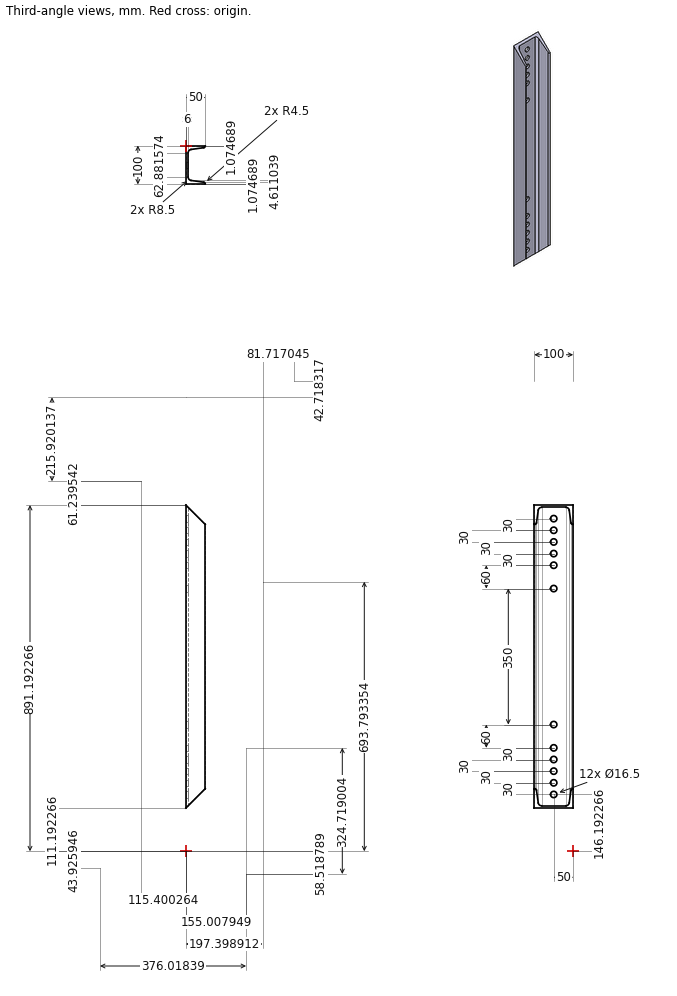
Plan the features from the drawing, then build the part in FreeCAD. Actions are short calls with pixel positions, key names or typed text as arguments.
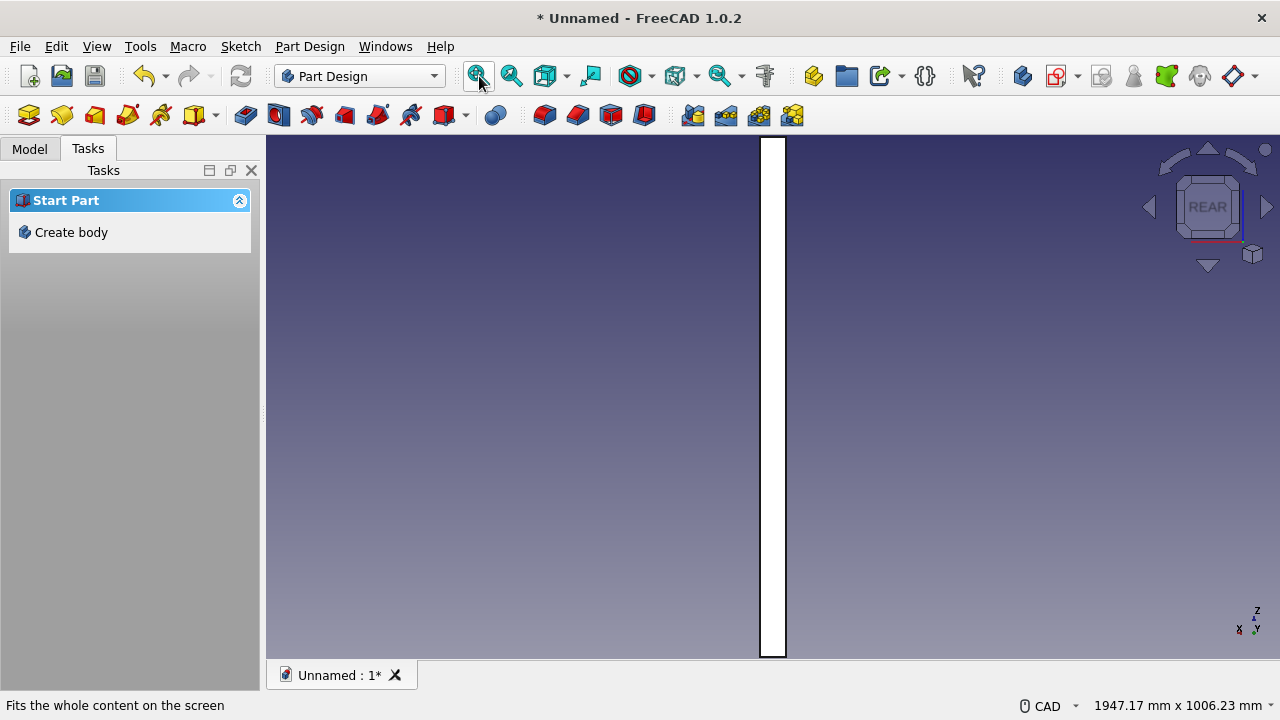
click(773, 173)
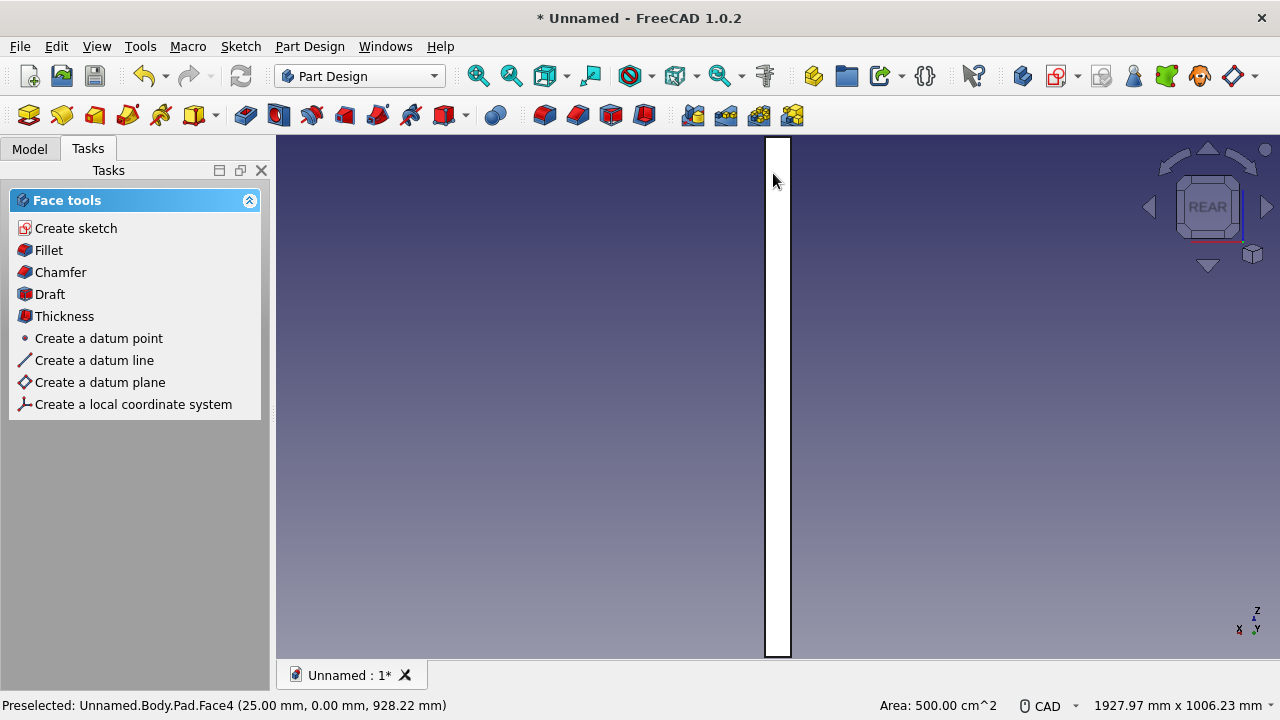
click(1056, 76)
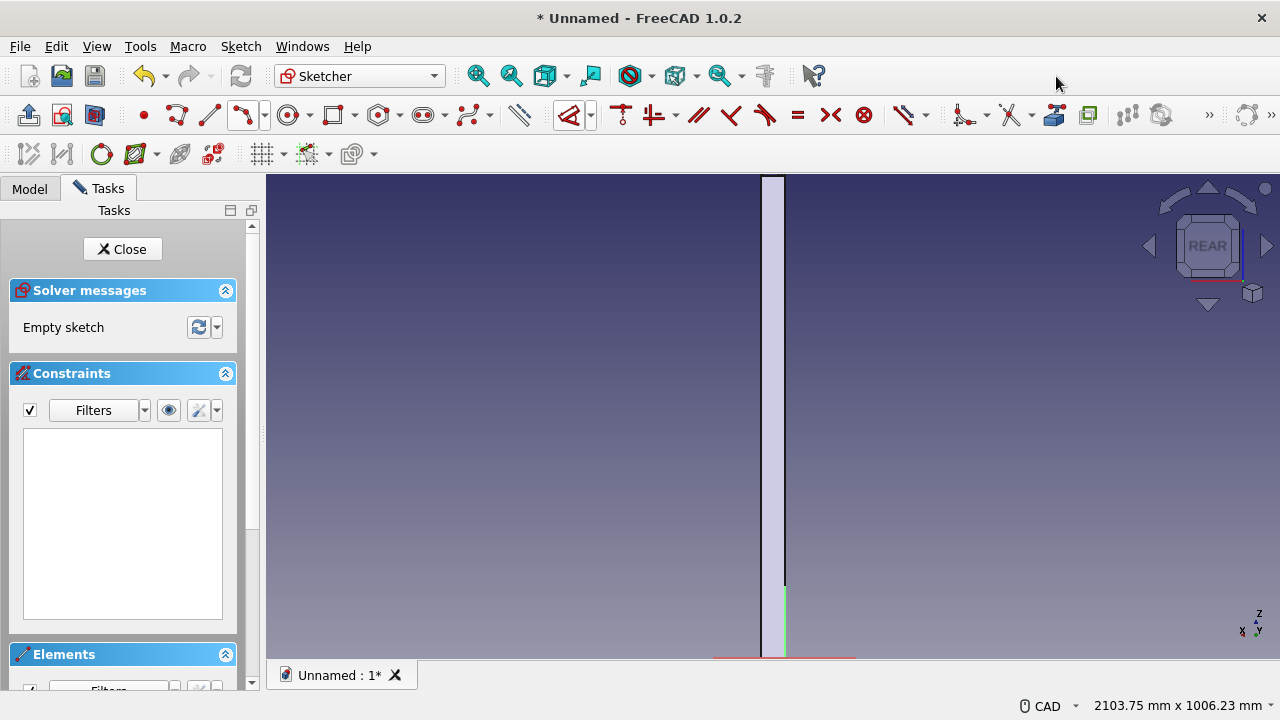
scroll(650, 446, down, 4)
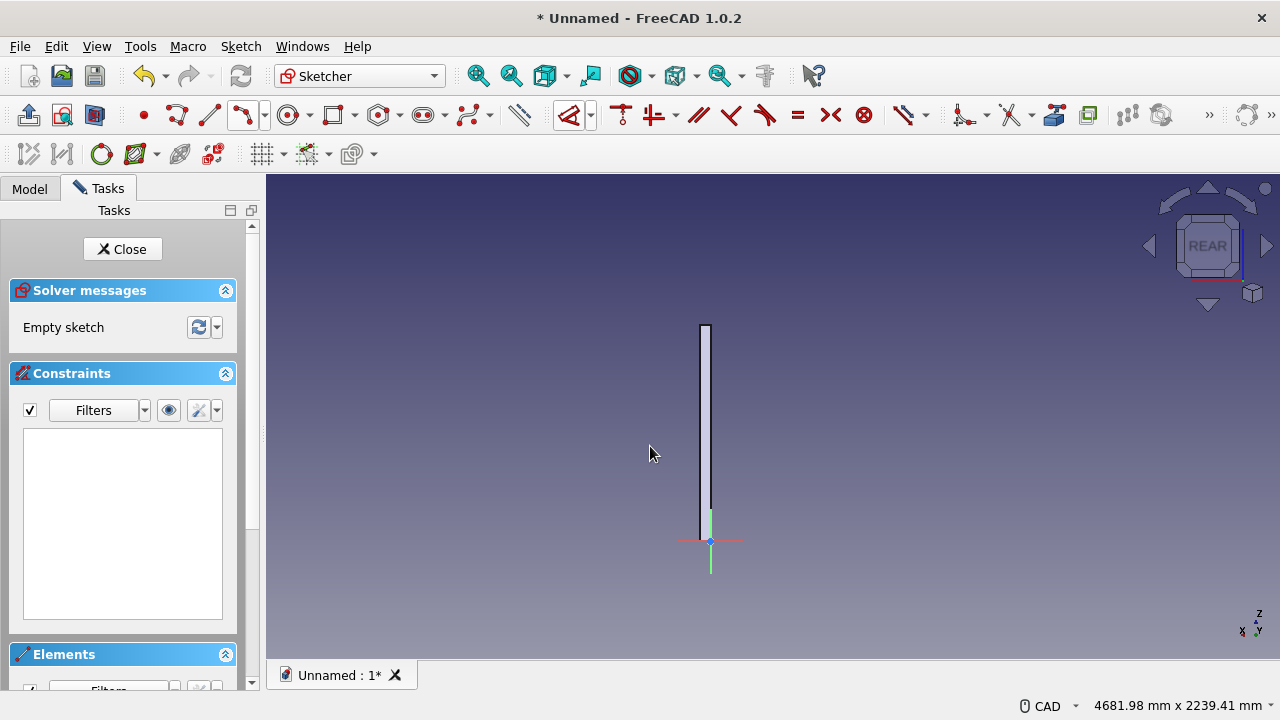
click(177, 116)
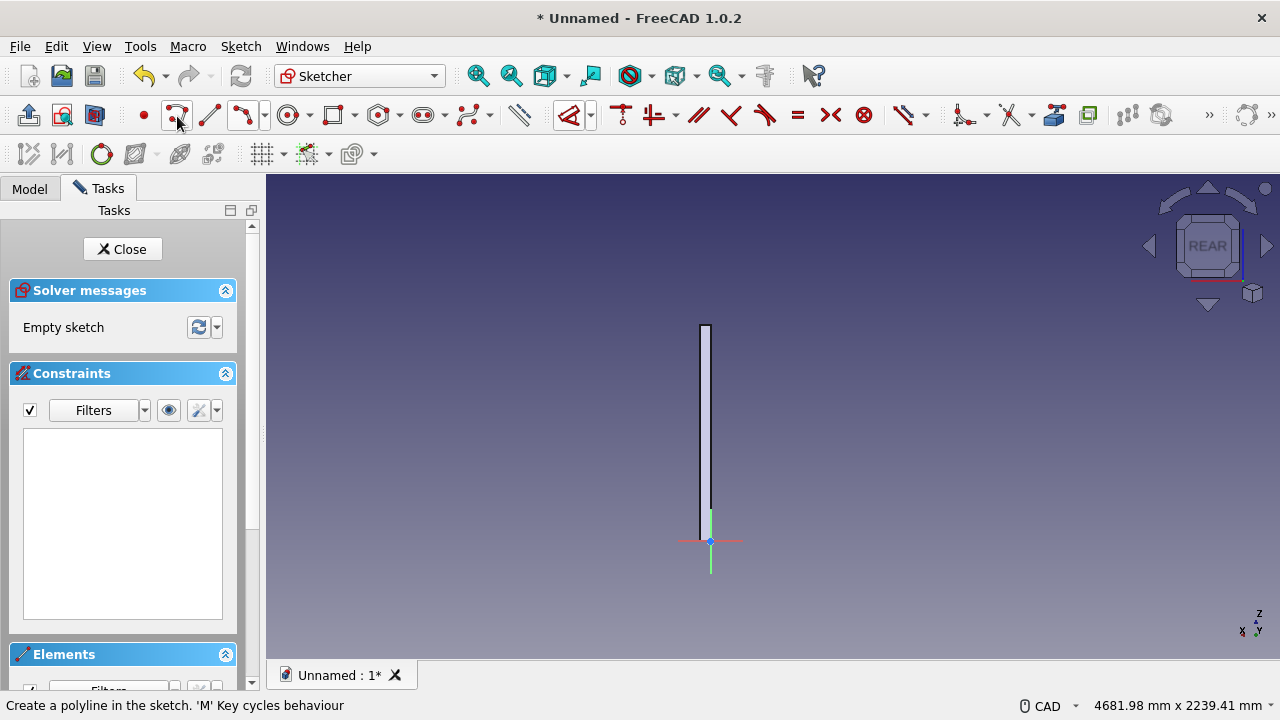
click(711, 517)
click(677, 484)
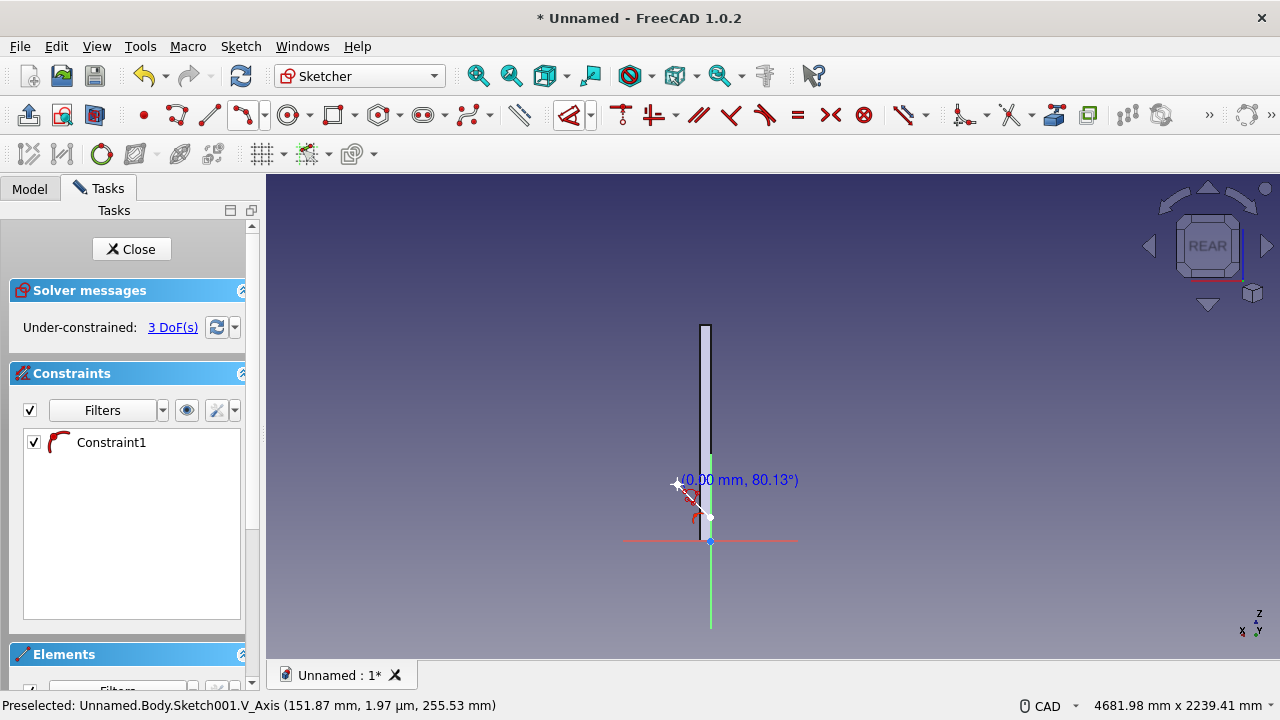
scroll(677, 554, up, 2)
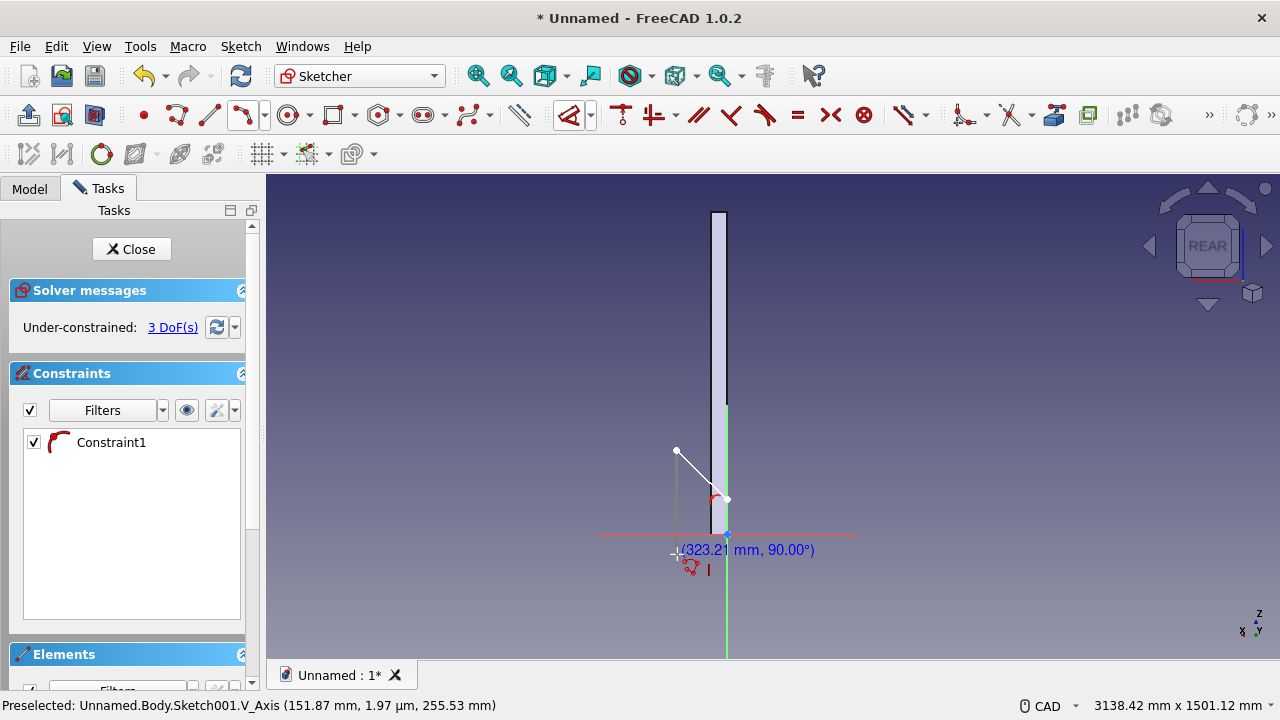
click(677, 554)
click(799, 547)
click(727, 500)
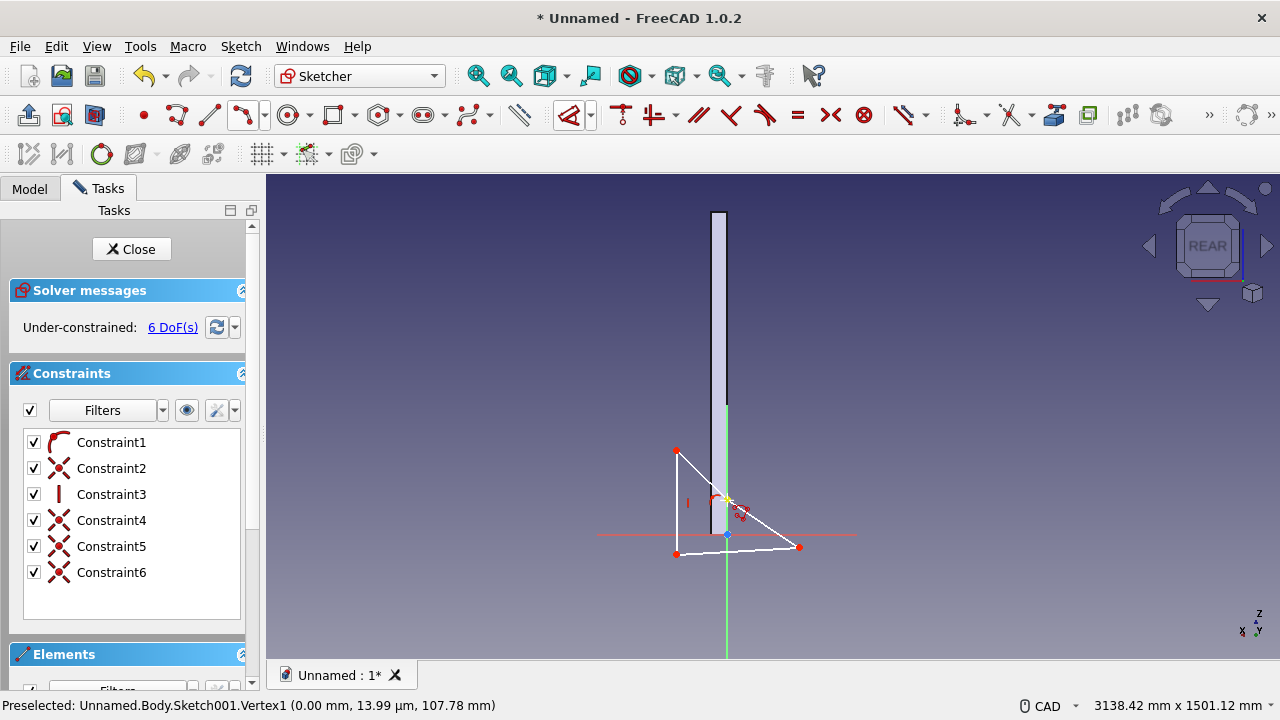
click(664, 311)
click(727, 247)
click(765, 227)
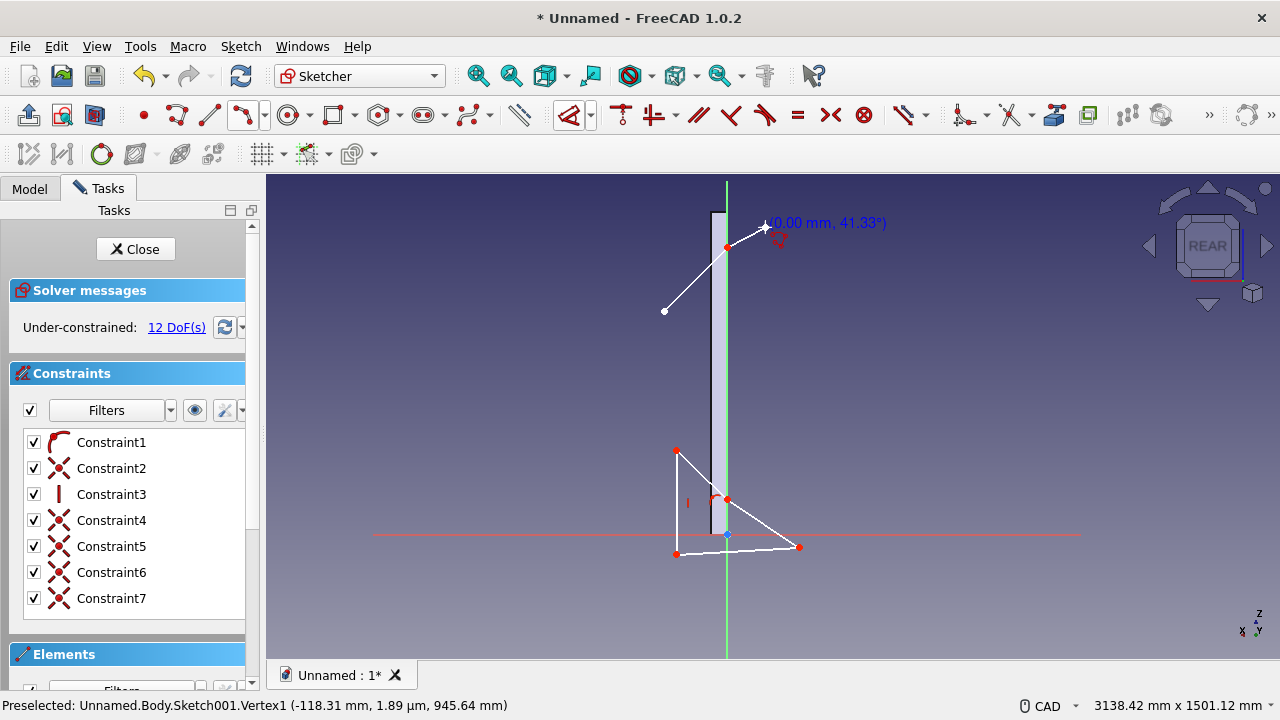
scroll(677, 555, down, 2)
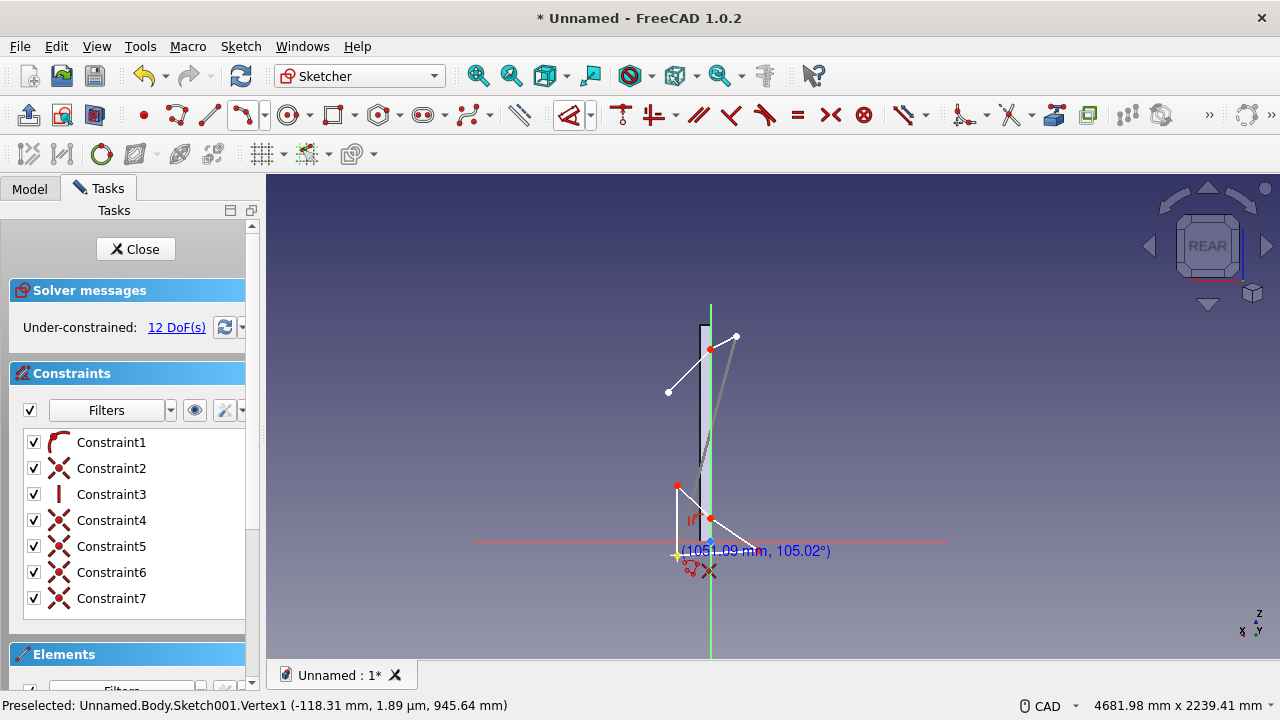
click(711, 289)
click(650, 279)
click(668, 392)
key(Escape)
key(Escape)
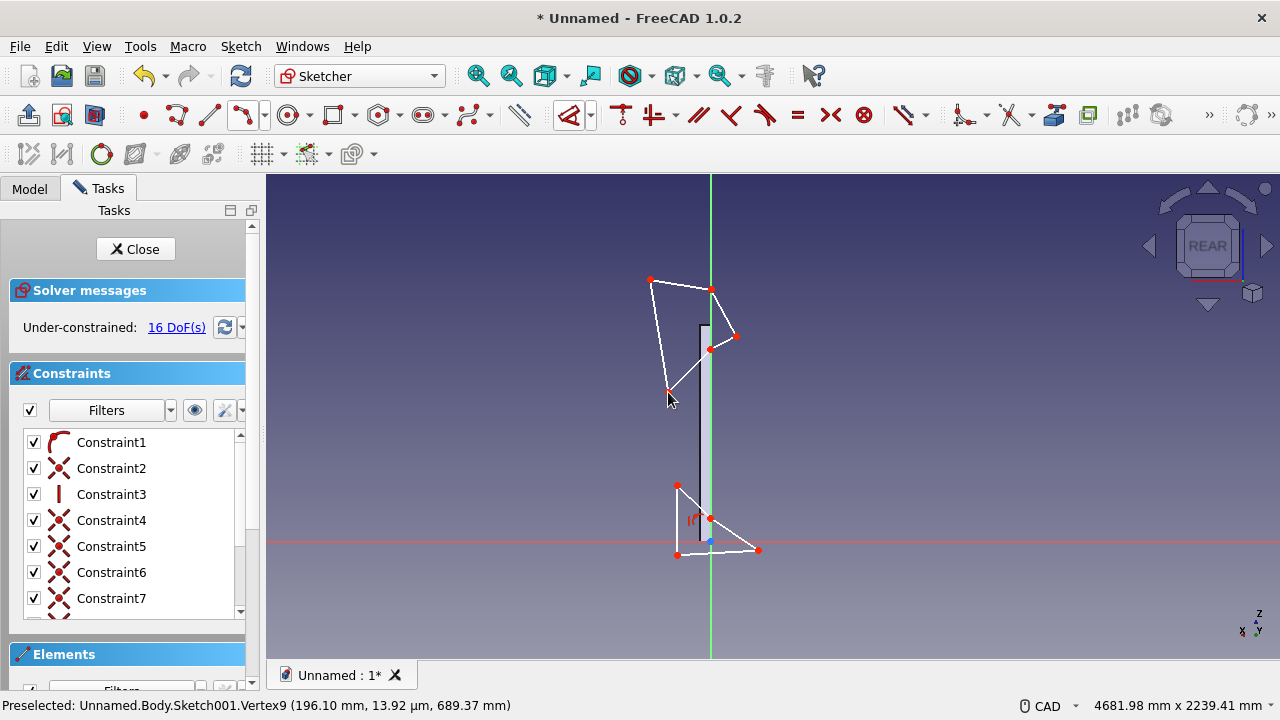
click(711, 349)